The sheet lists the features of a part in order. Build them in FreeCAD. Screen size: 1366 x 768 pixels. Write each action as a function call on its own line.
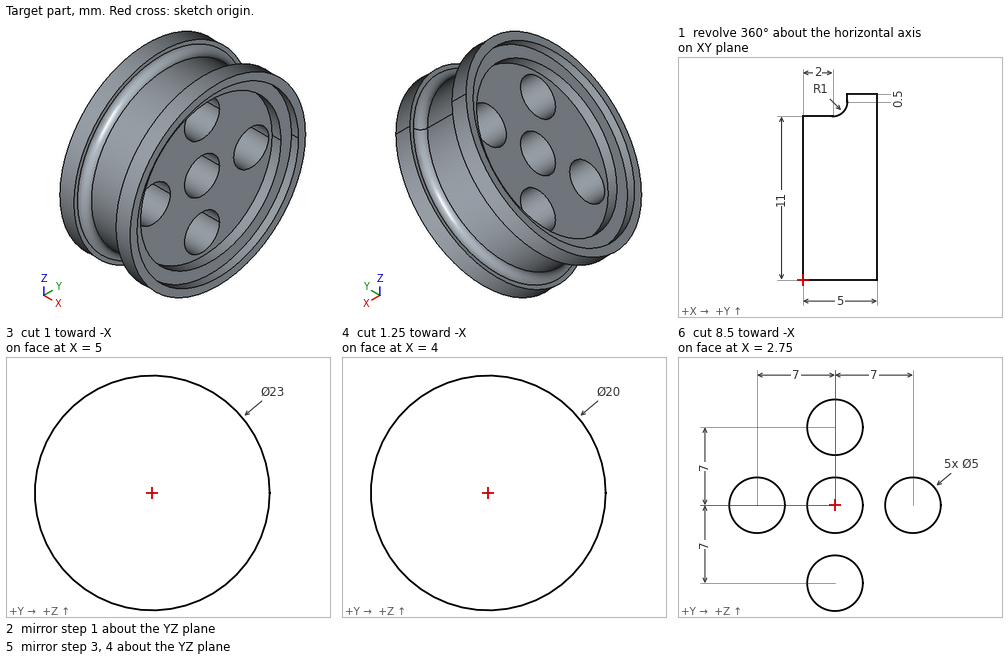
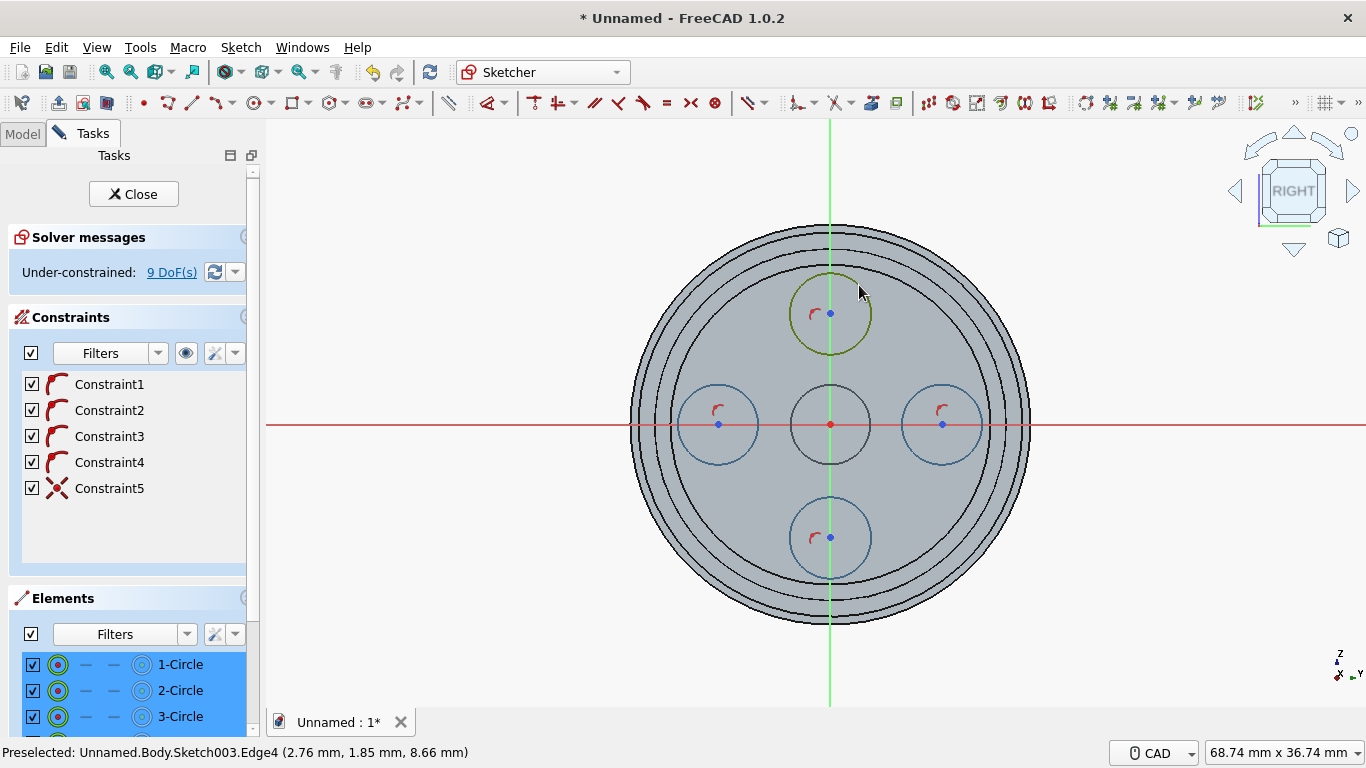
click(858, 396)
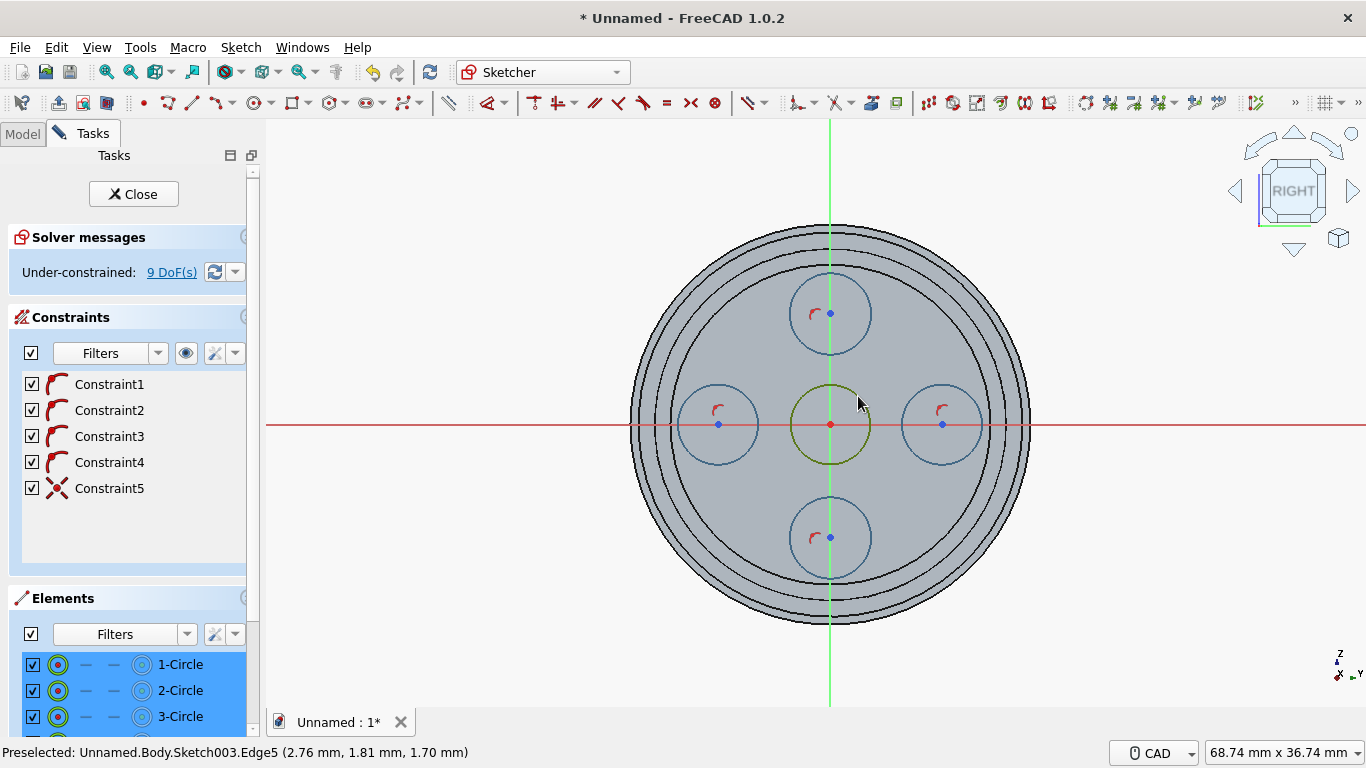
click(668, 104)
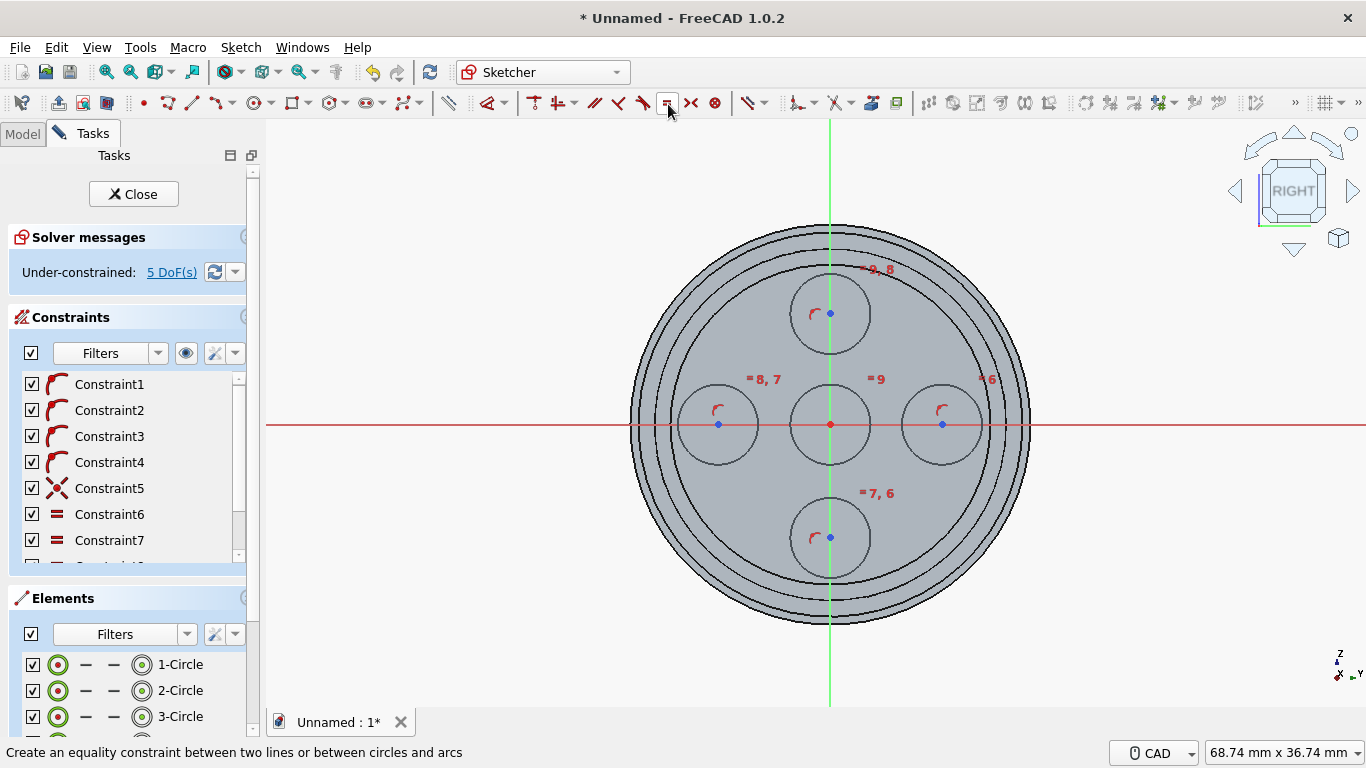
click(488, 104)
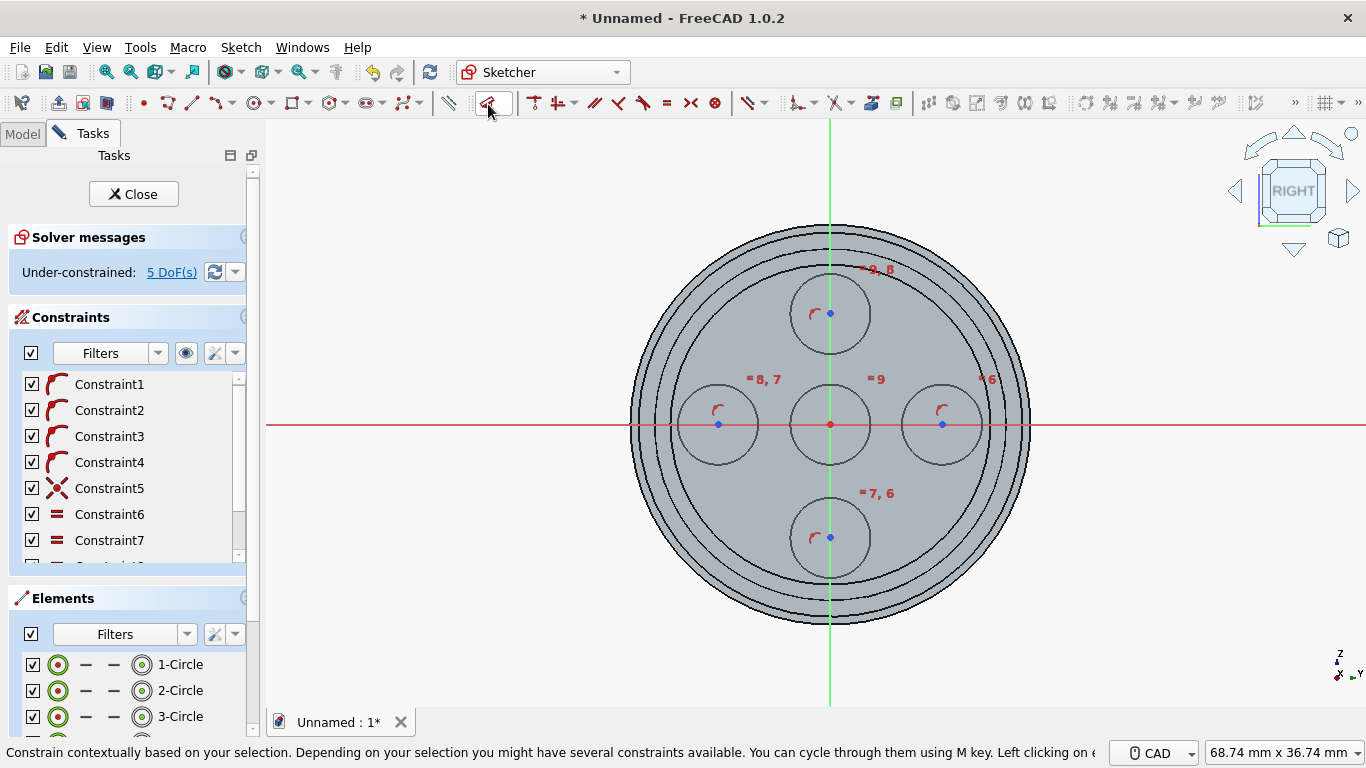
click(970, 396)
click(992, 373)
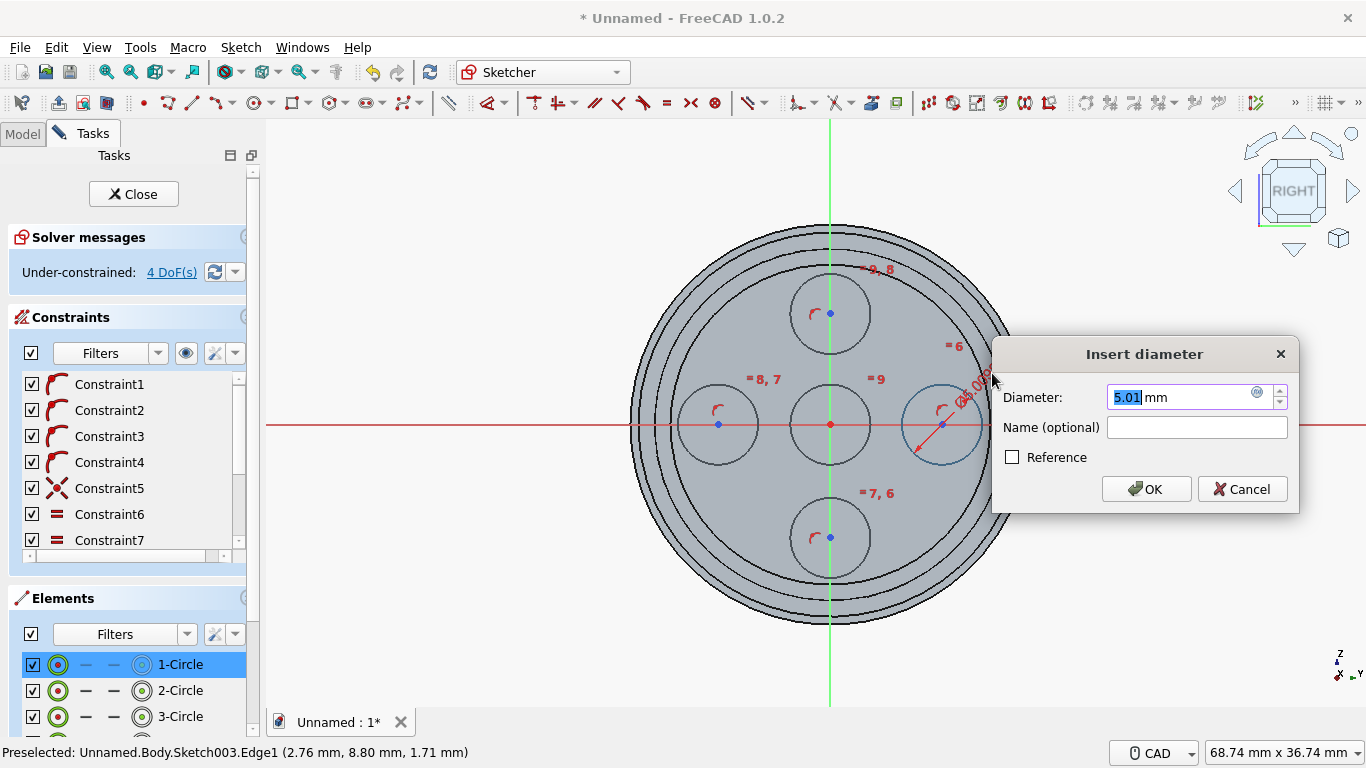
text(5)
key(Return)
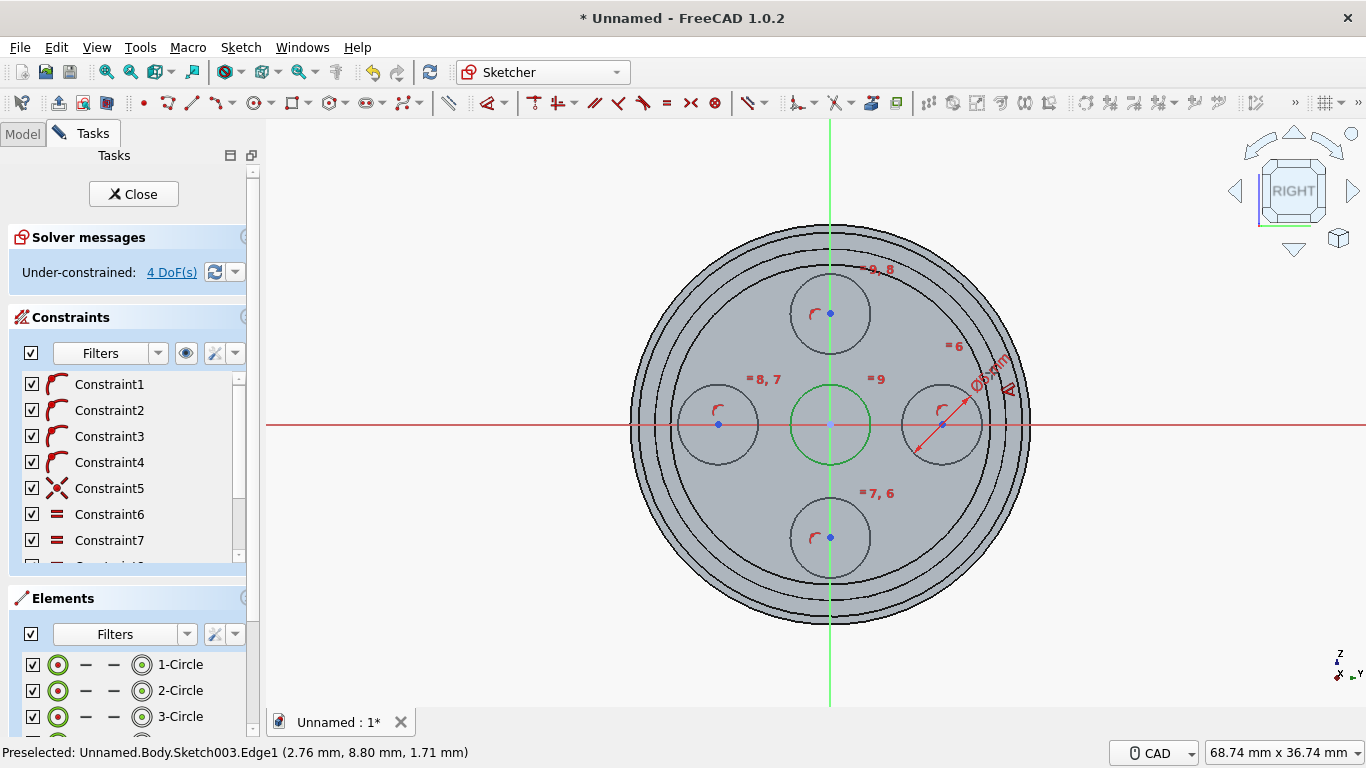
click(942, 425)
click(886, 459)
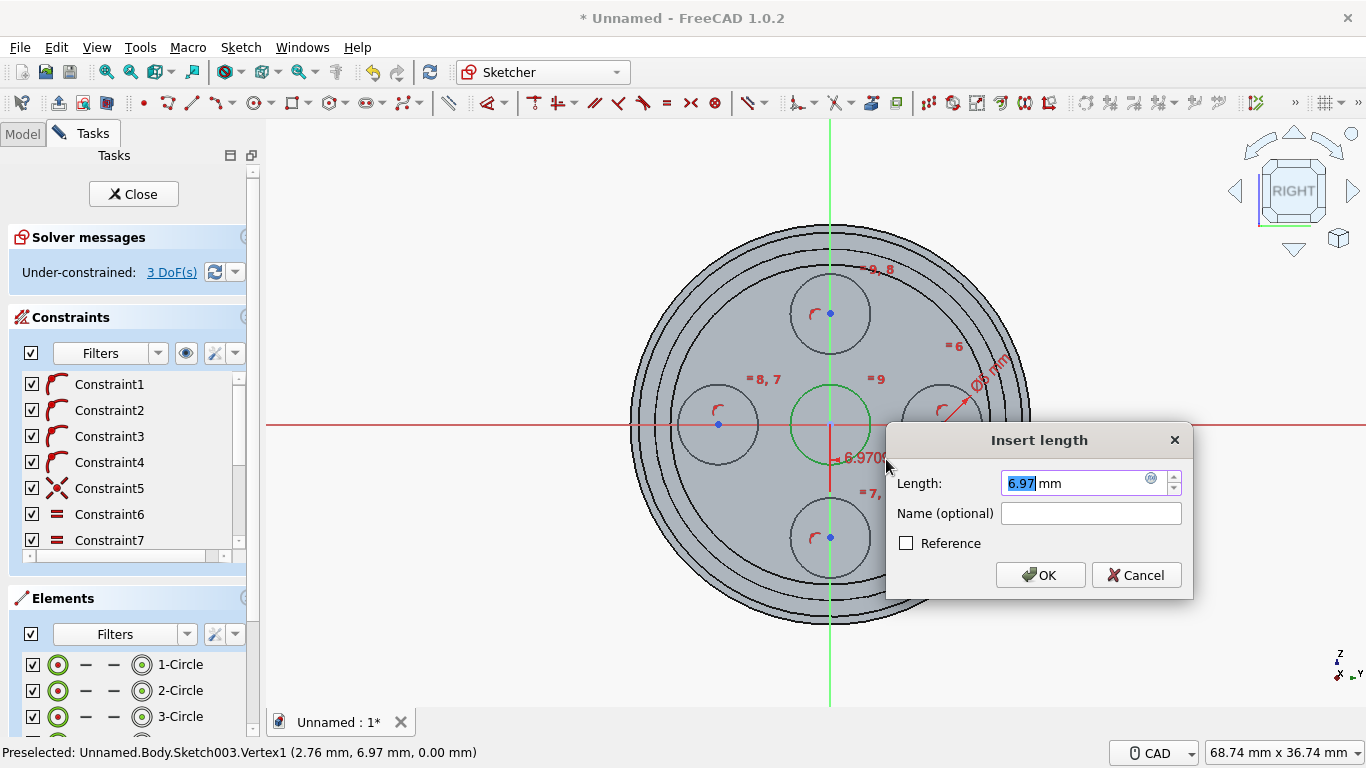
text(7)
key(Return)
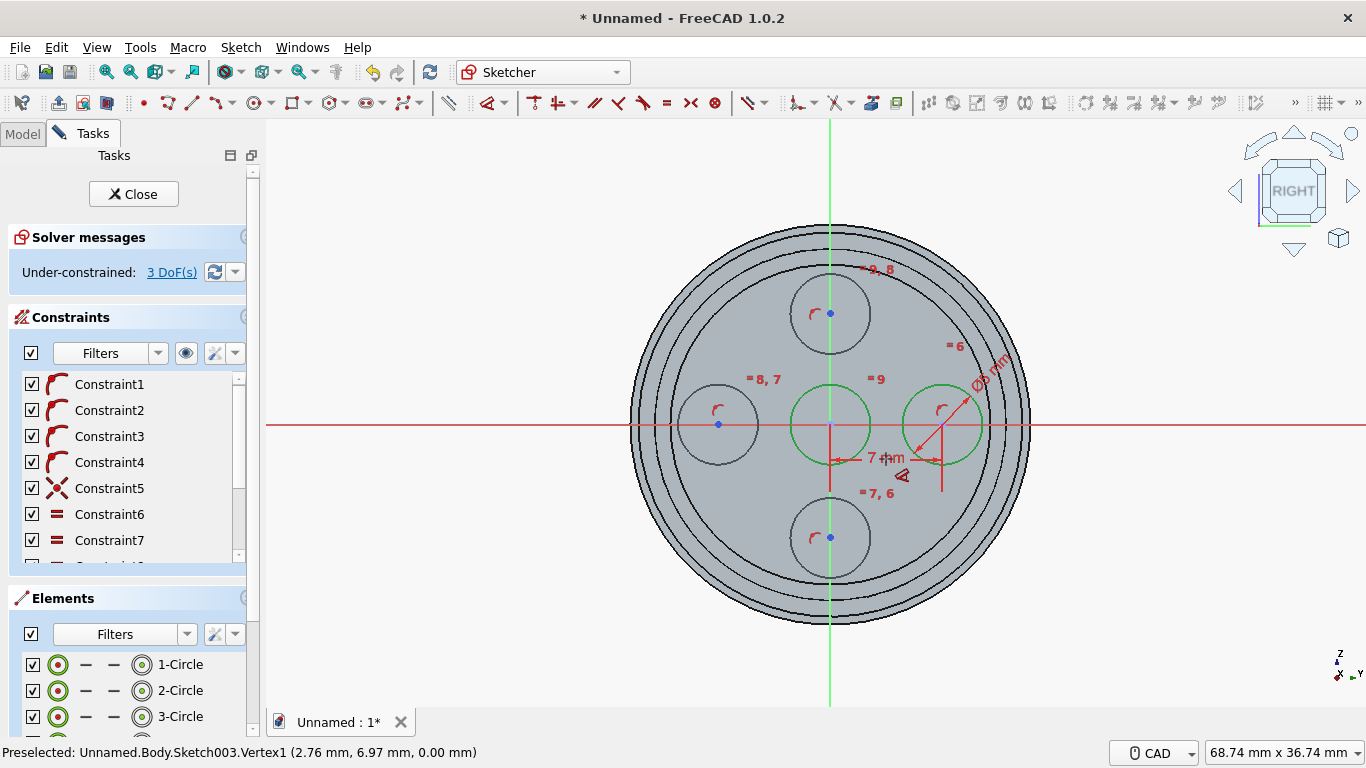
click(830, 538)
click(864, 481)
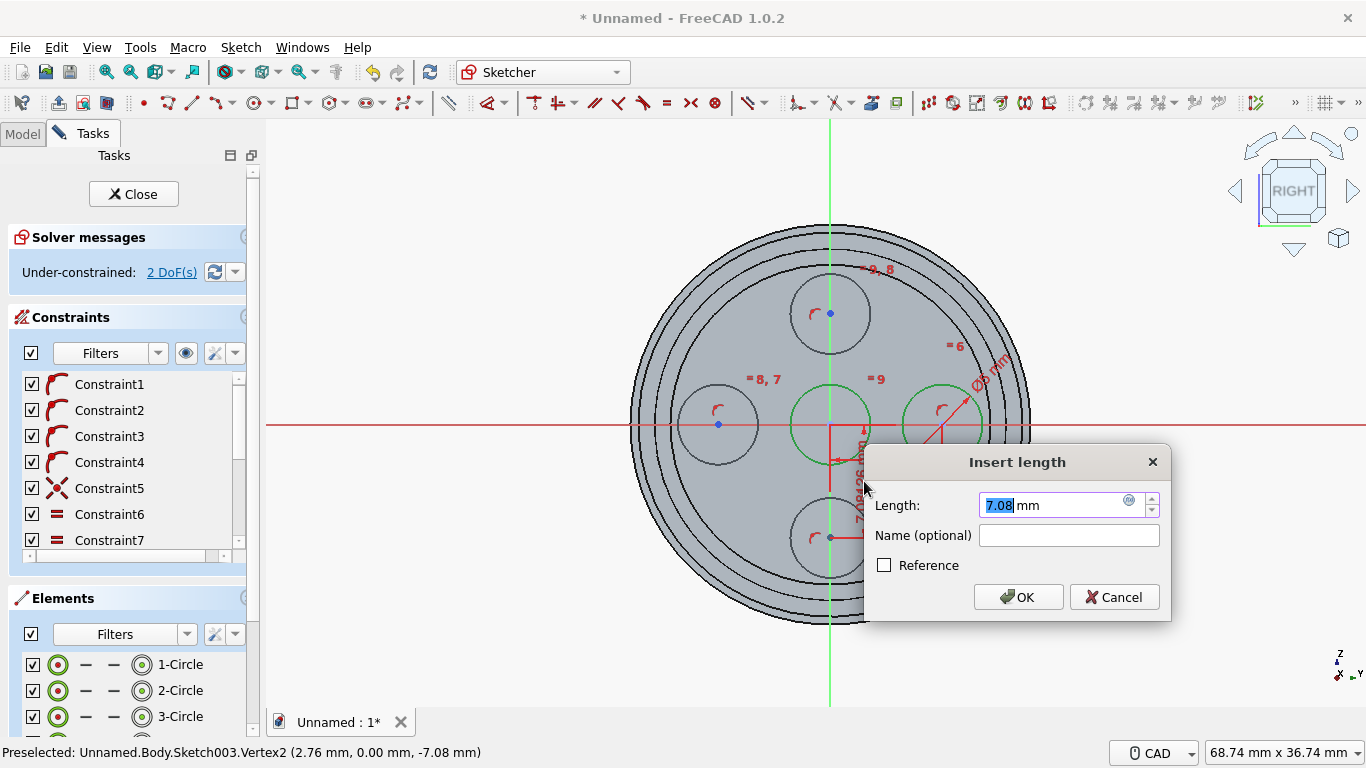
text(7)
key(Return)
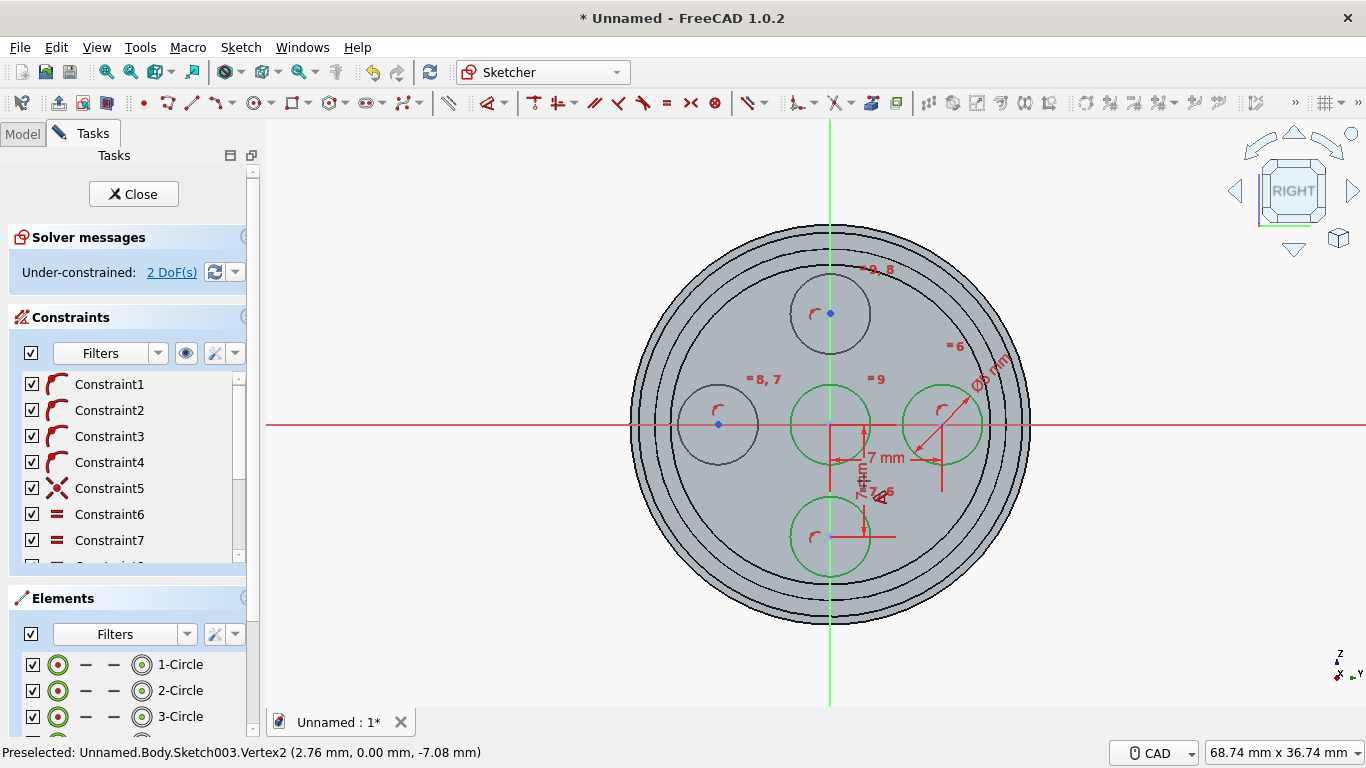
click(718, 425)
click(774, 459)